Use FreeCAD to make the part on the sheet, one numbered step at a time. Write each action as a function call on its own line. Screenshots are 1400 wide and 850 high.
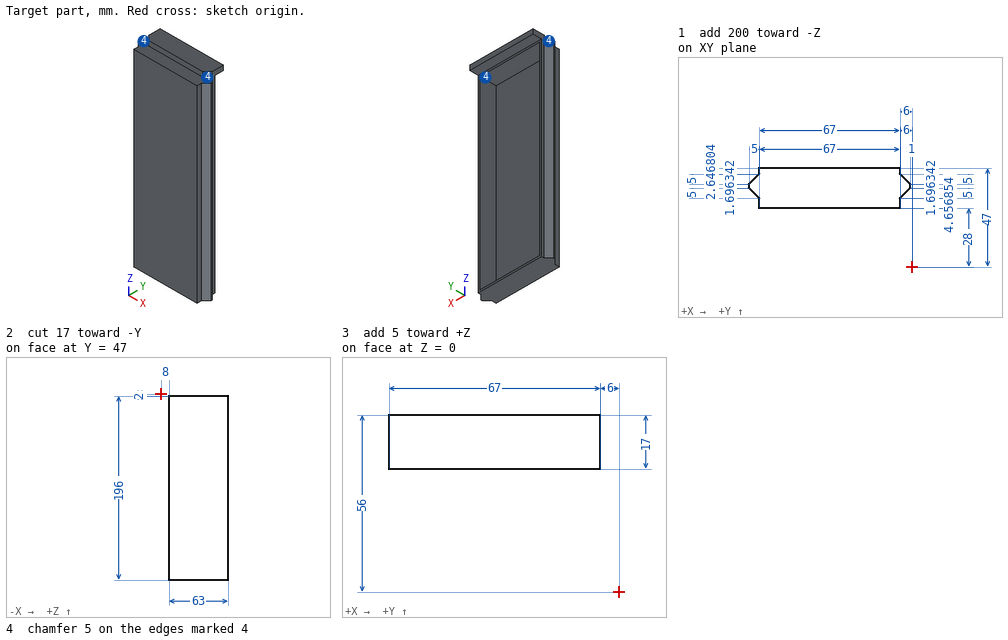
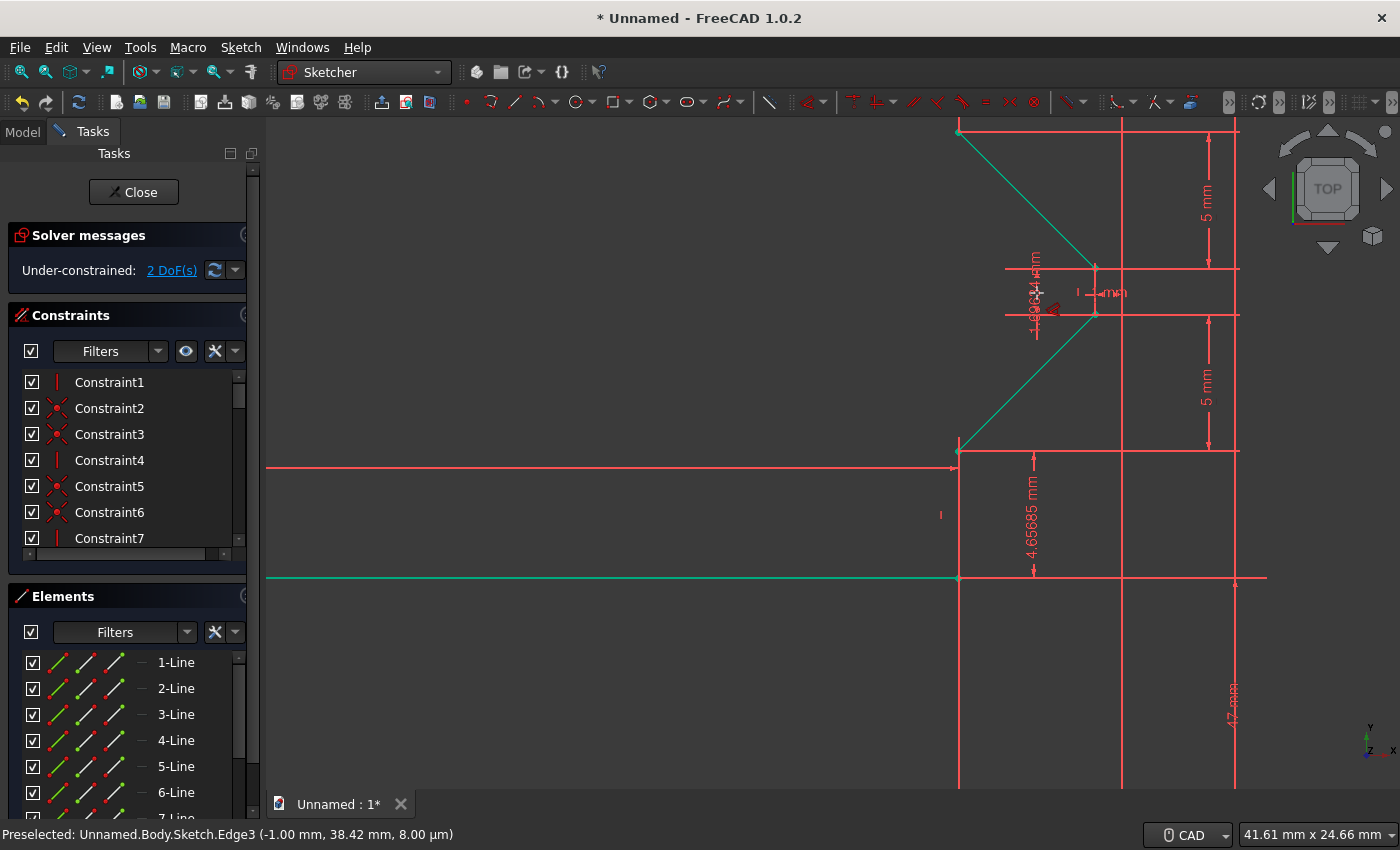
scroll(1068, 346, down, 6)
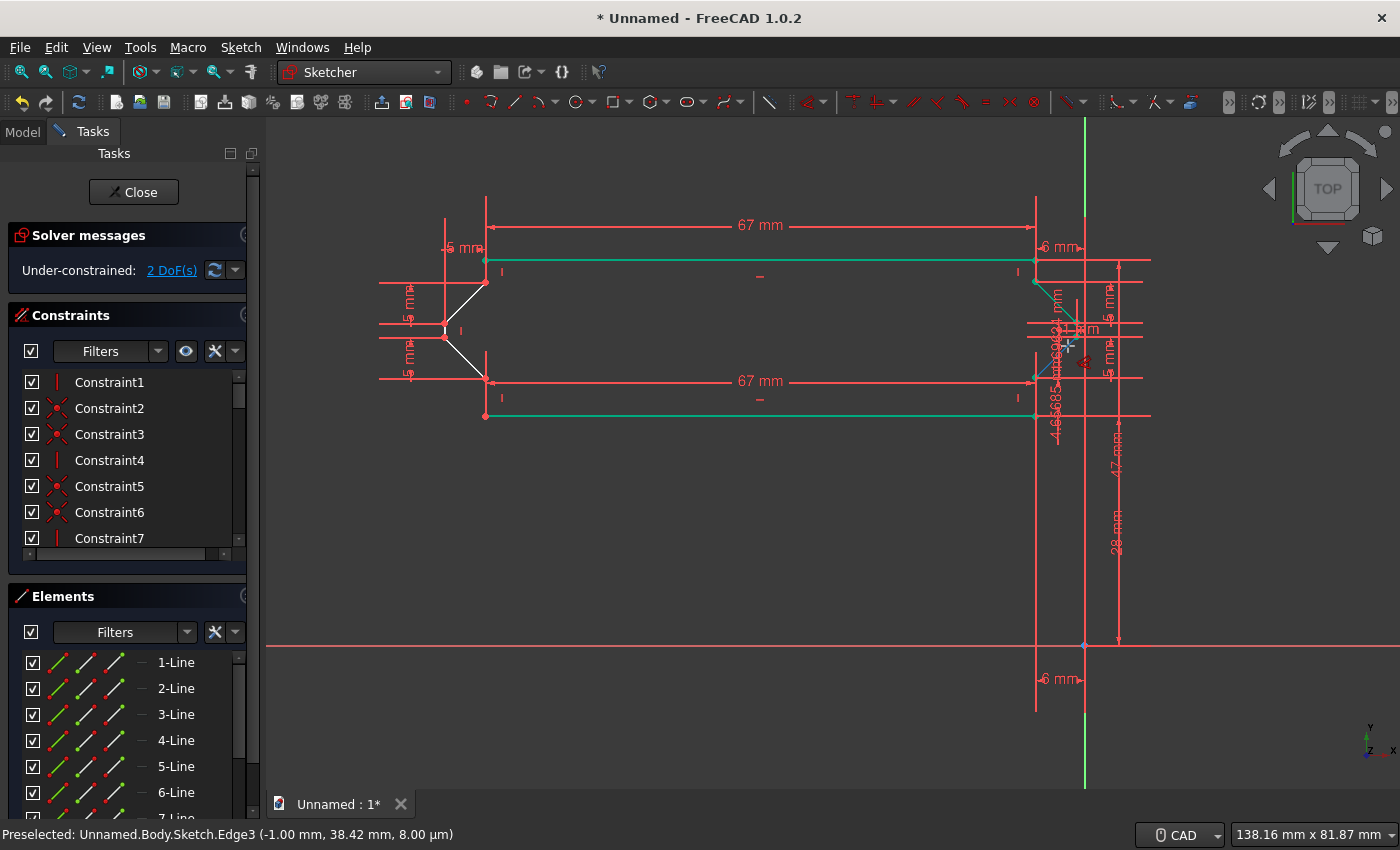
scroll(486, 267, up, 4)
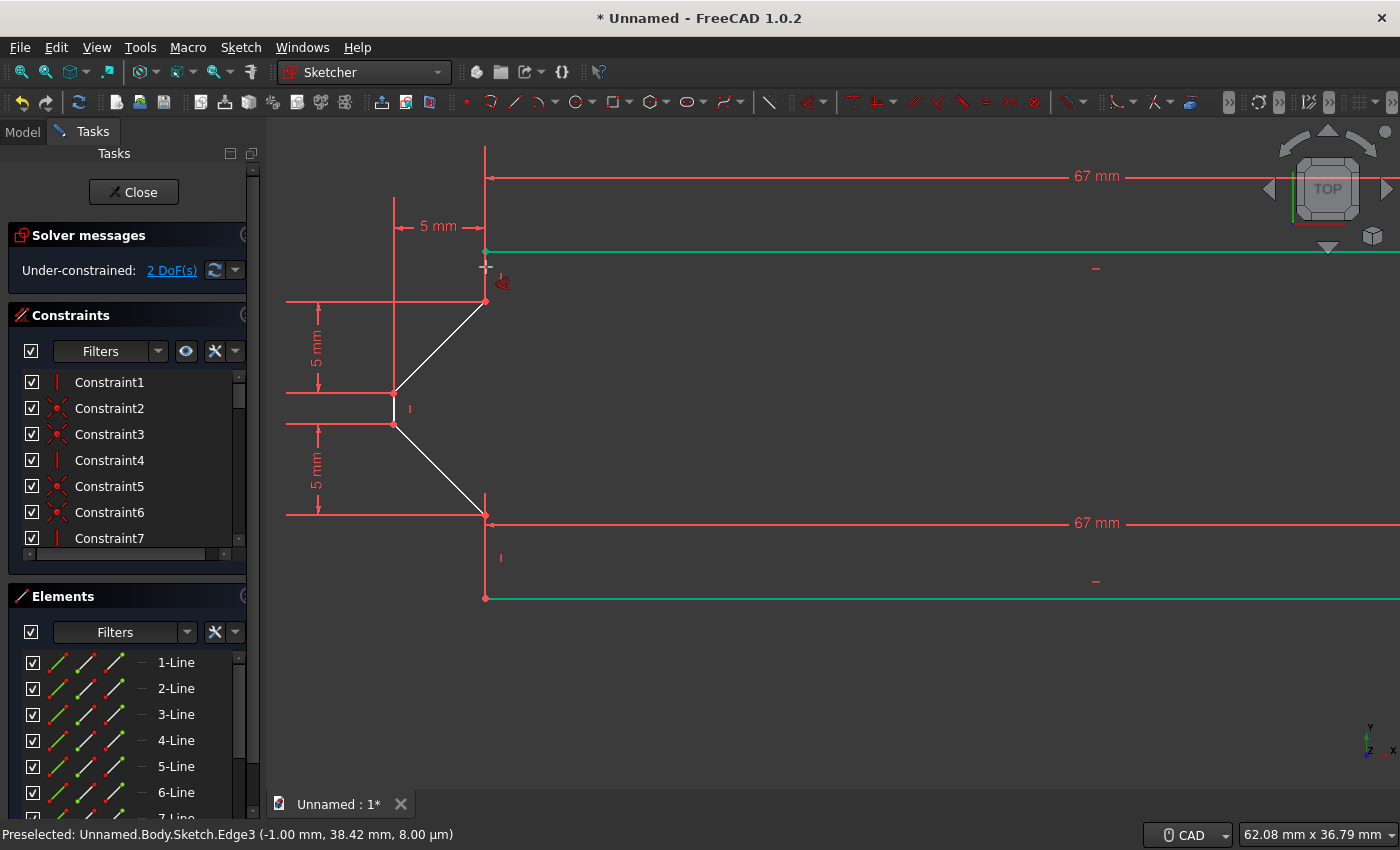
click(485, 267)
click(451, 277)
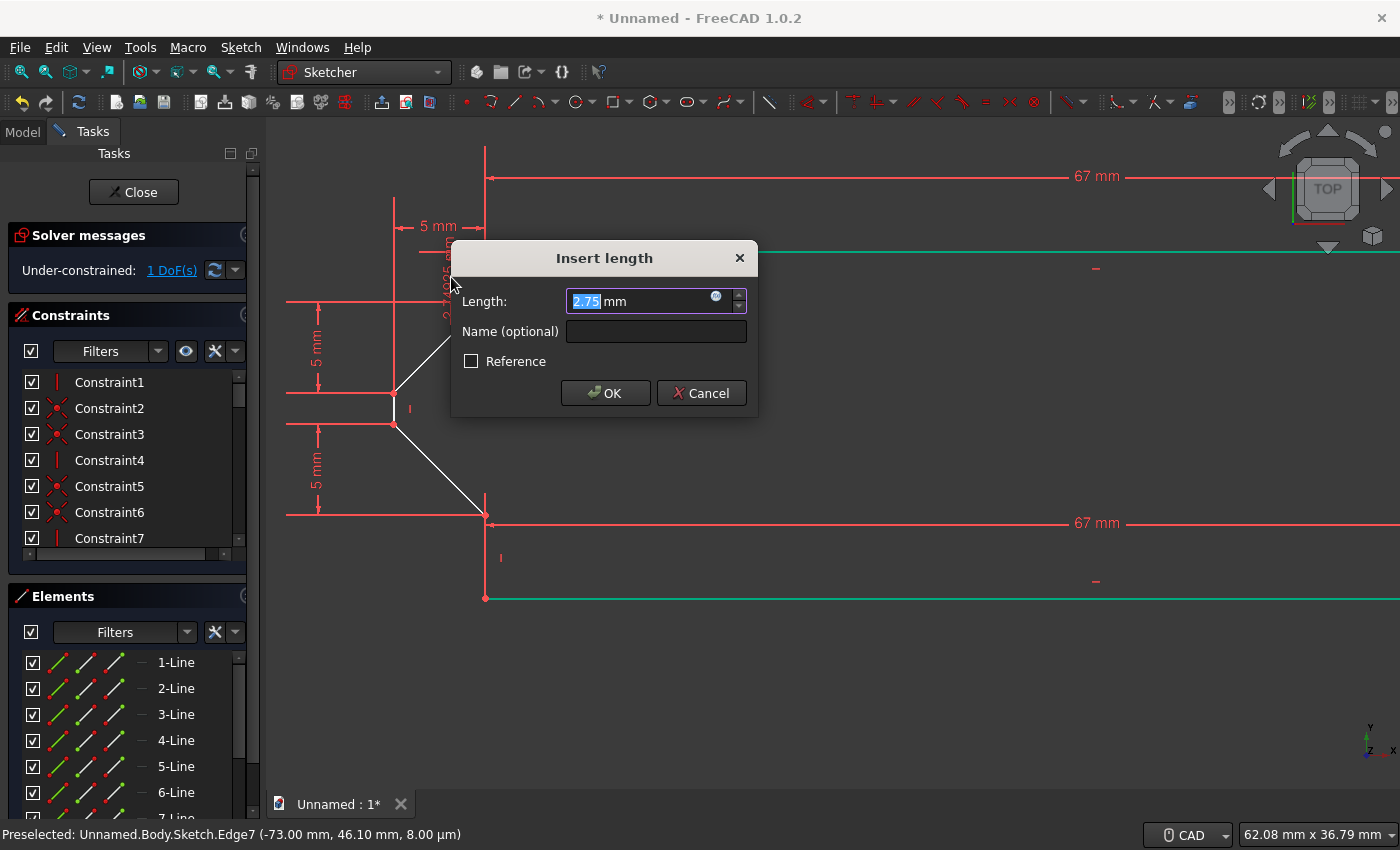
text(2.646804)
key(Return)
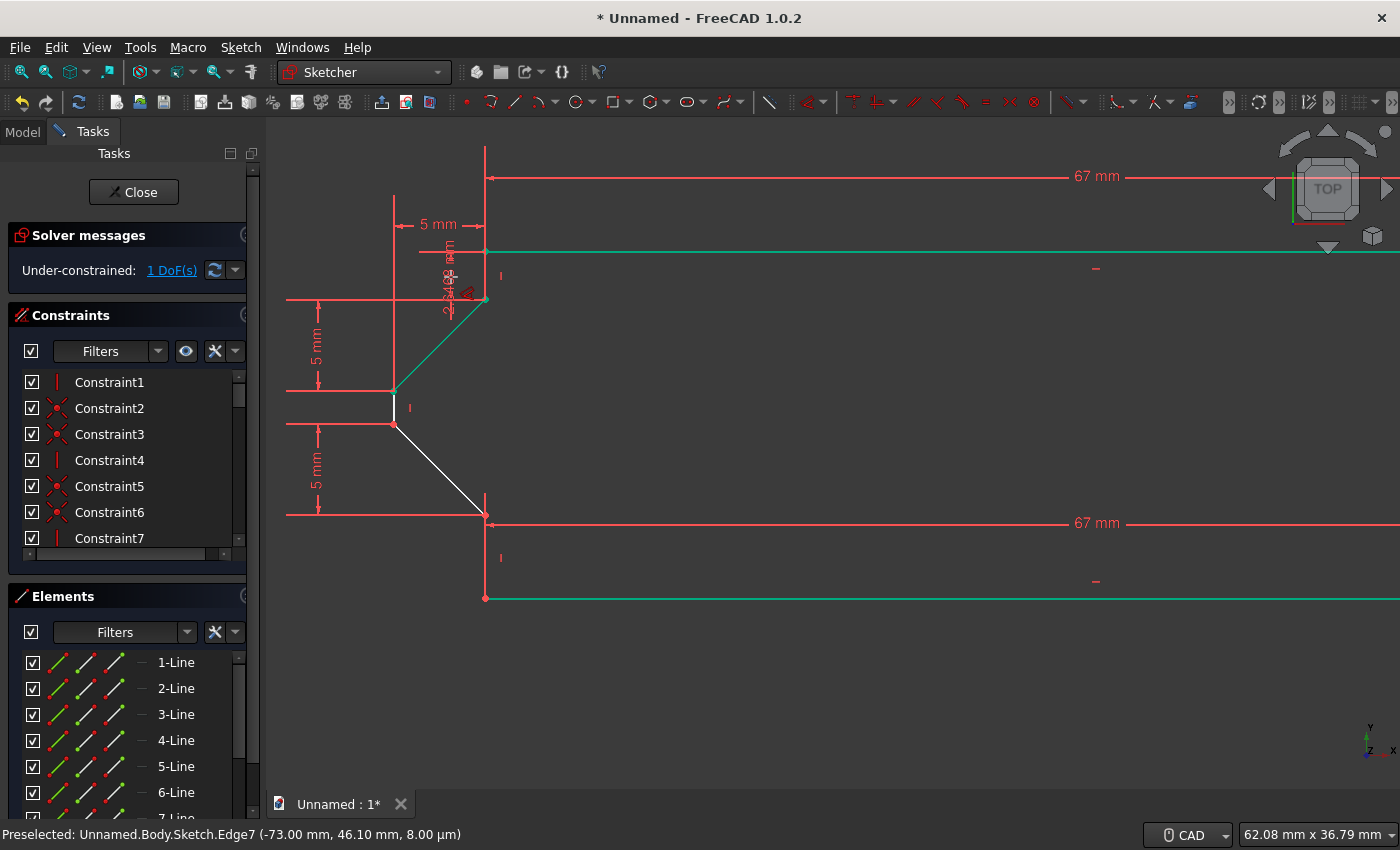
scroll(394, 401, up, 2)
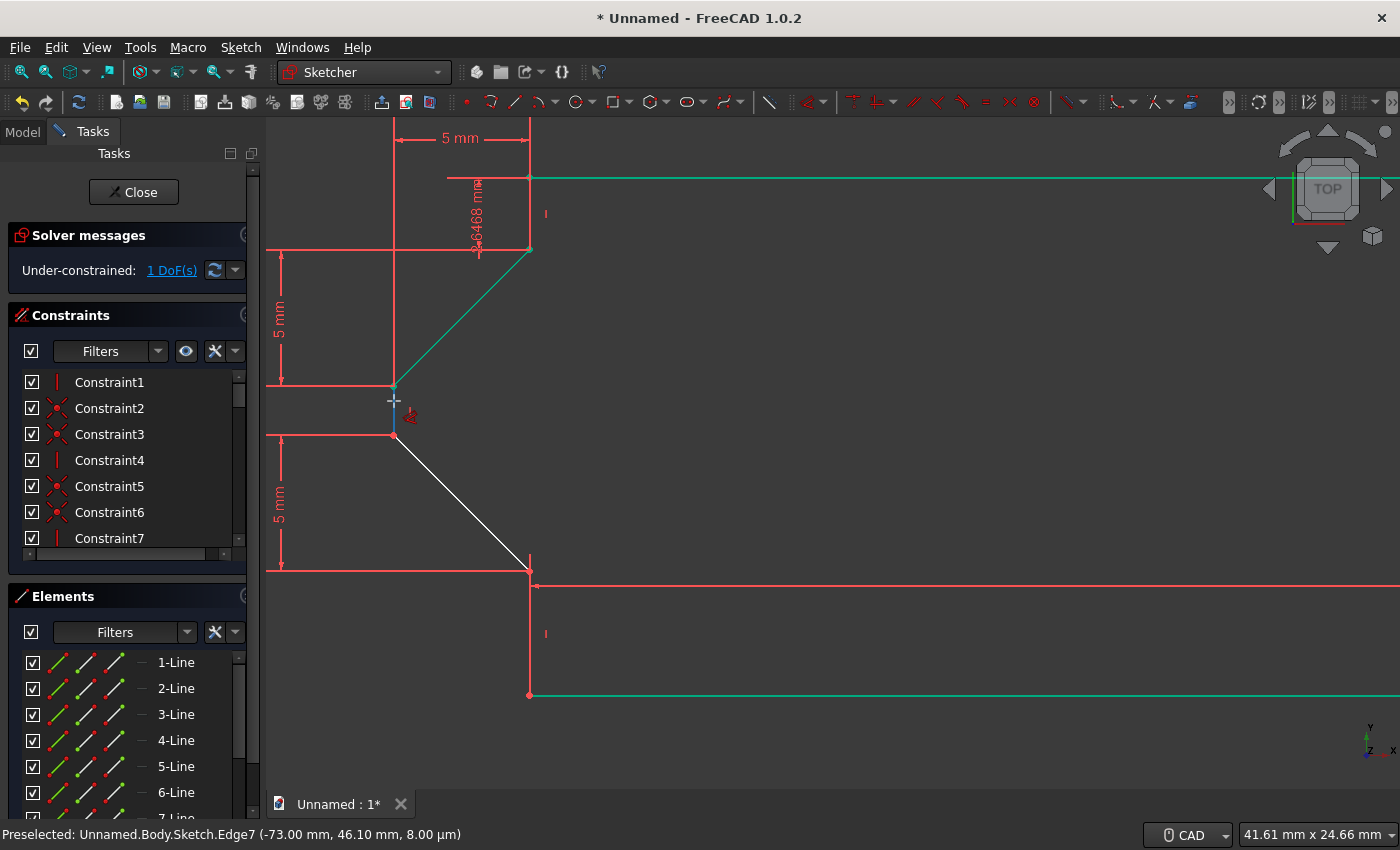
click(394, 401)
click(360, 411)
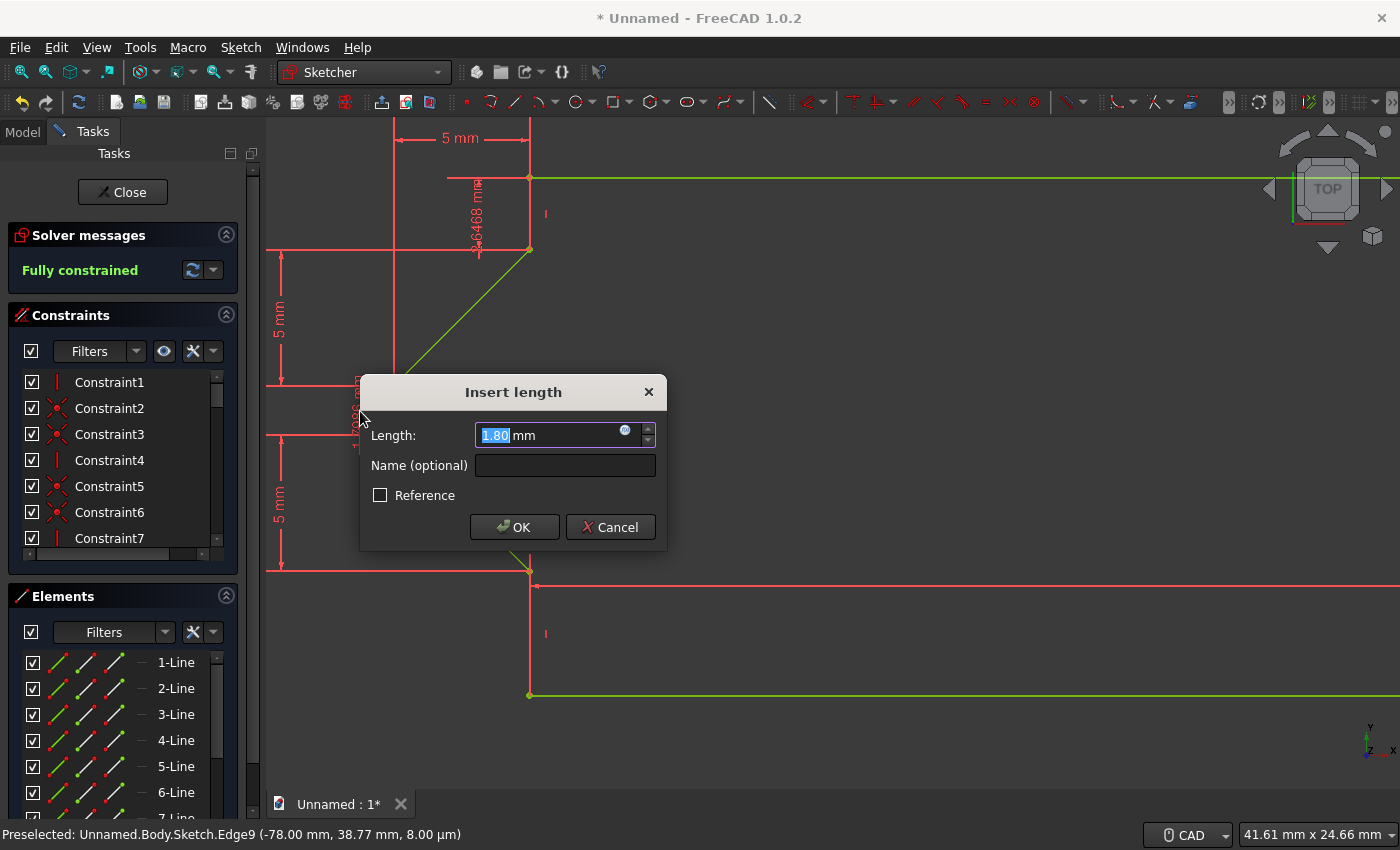
text(1.696342)
key(Return)
key(Escape)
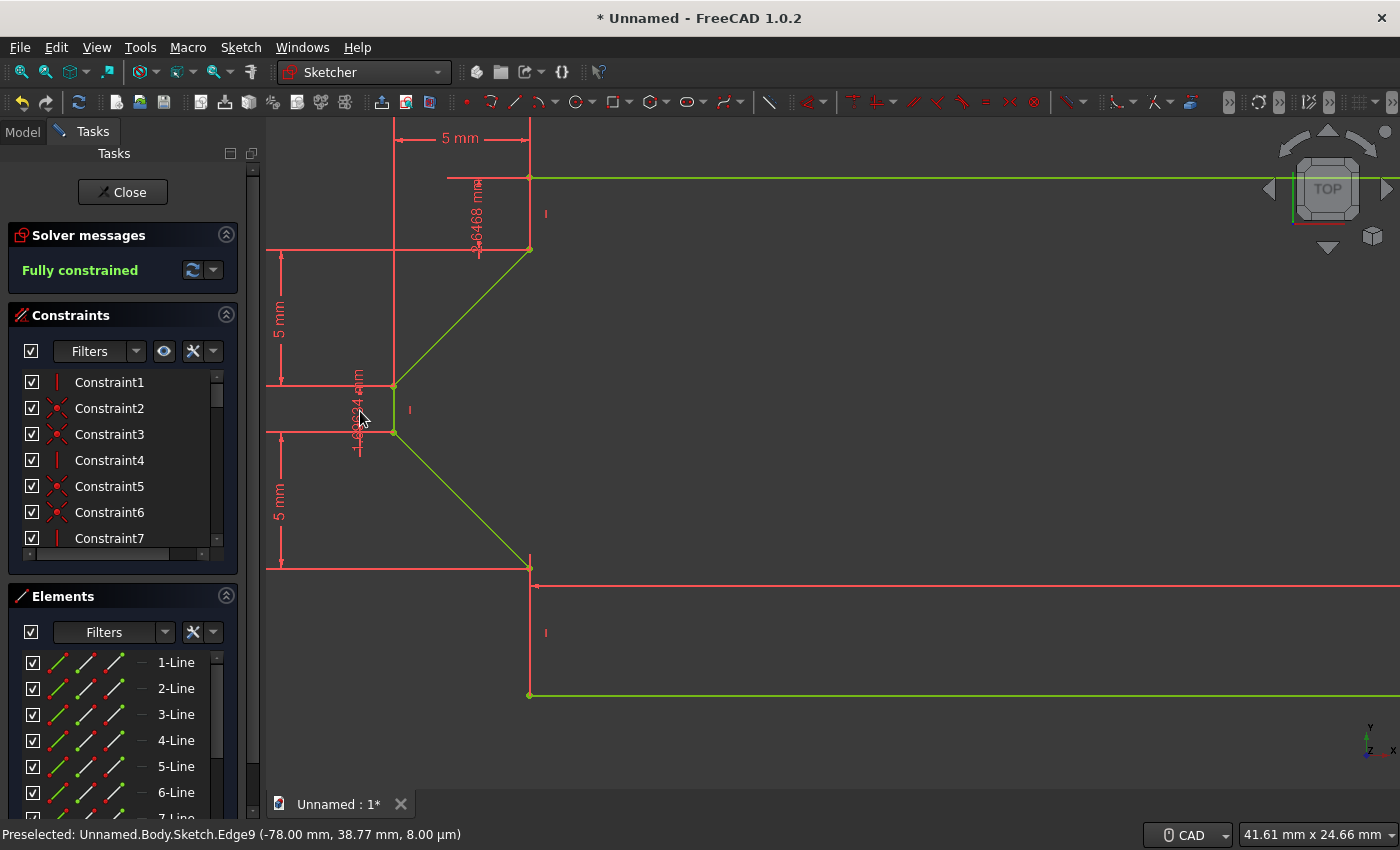
click(123, 192)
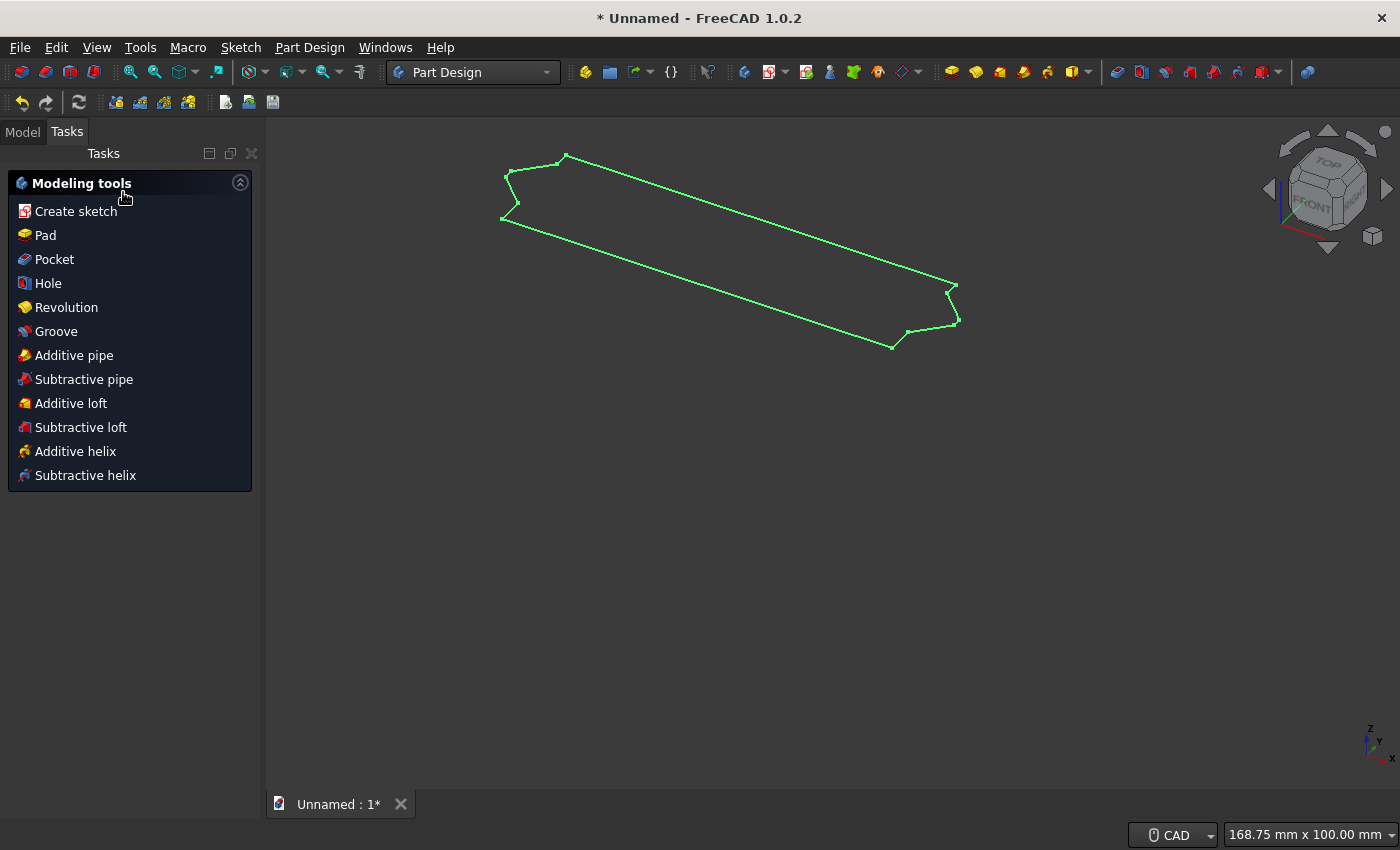
click(952, 72)